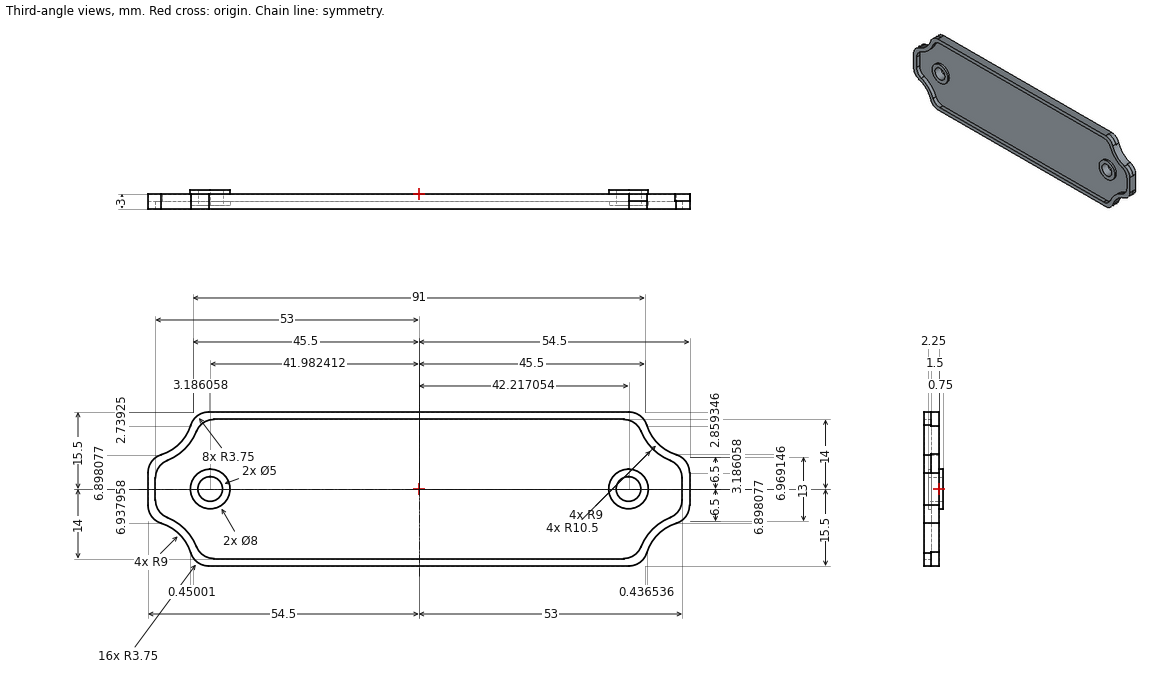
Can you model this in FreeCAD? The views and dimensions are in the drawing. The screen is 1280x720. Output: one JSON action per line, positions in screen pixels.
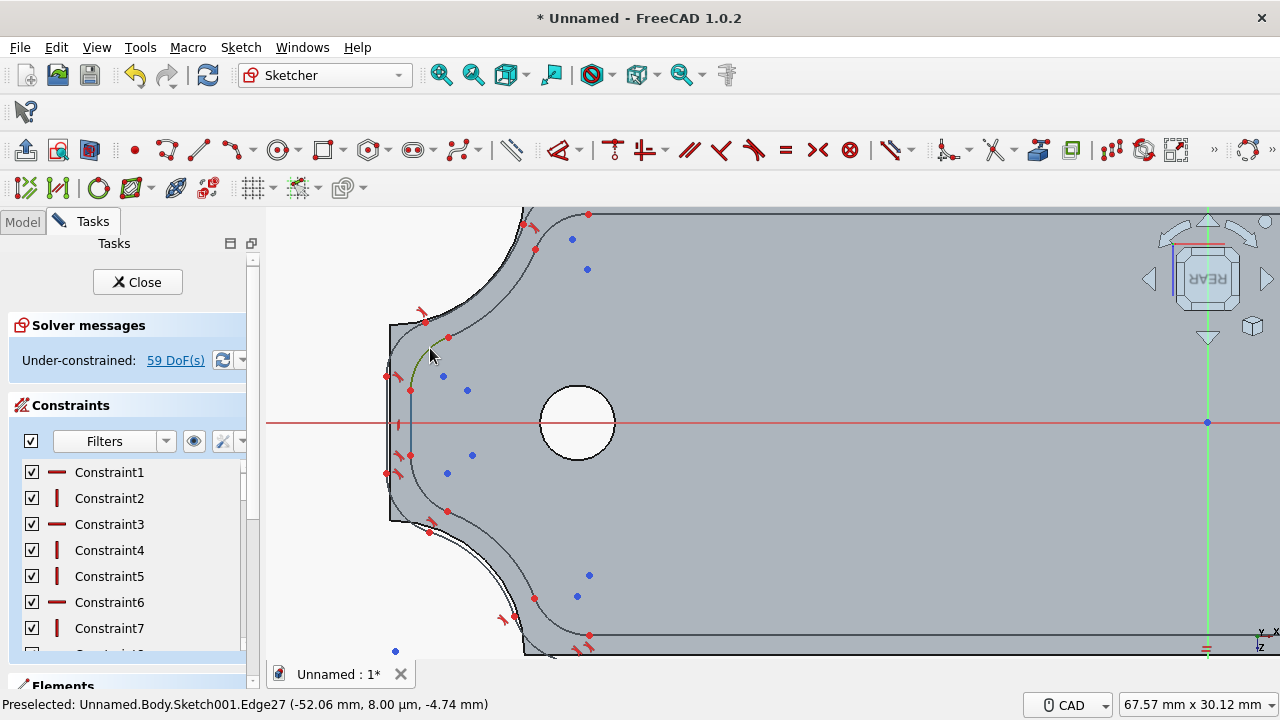
{"action": "left_click", "coordinate": [754, 150]}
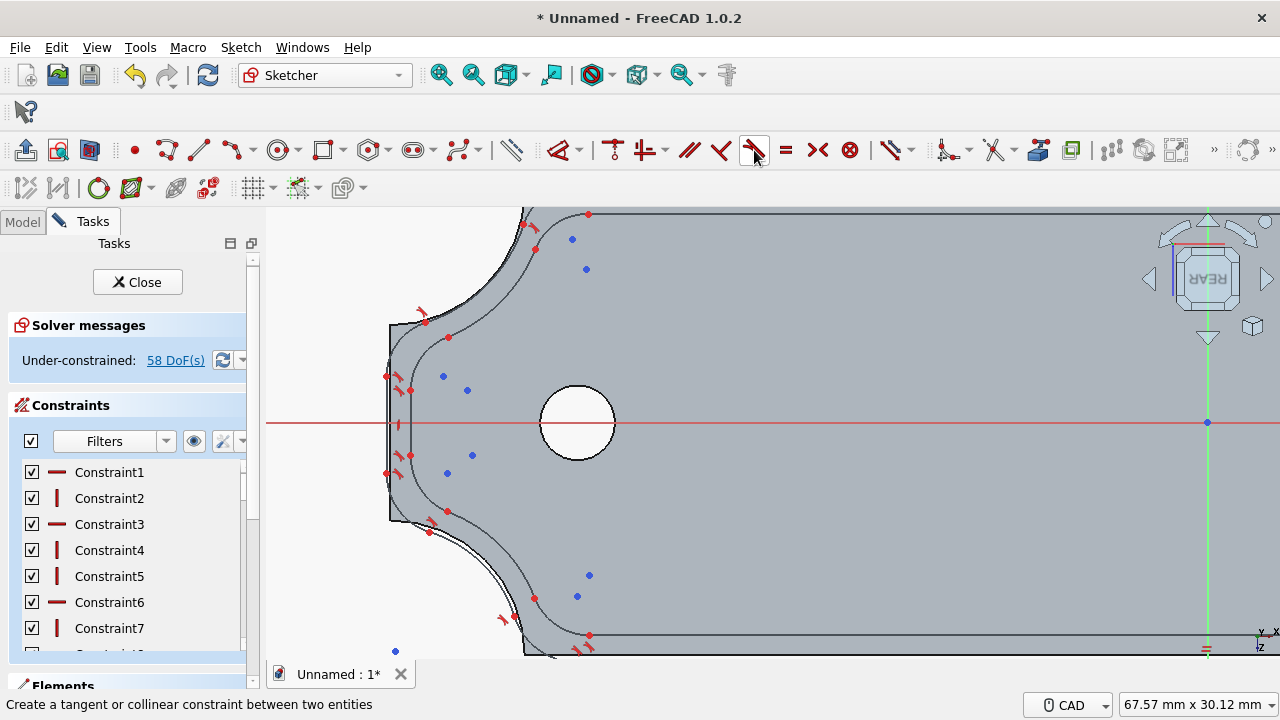
{"action": "scroll", "coordinate": [412, 439], "scroll_direction": "down", "scroll_amount": 5}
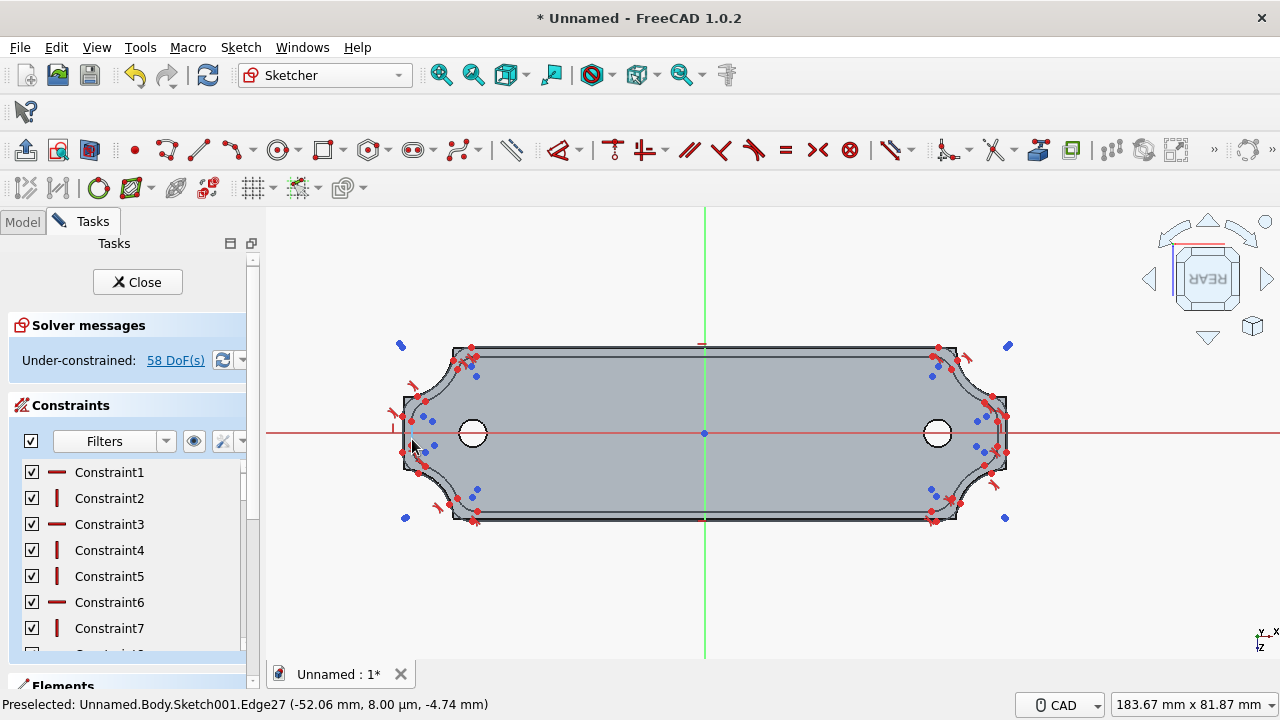
{"action": "scroll", "coordinate": [614, 357], "scroll_direction": "up", "scroll_amount": 2}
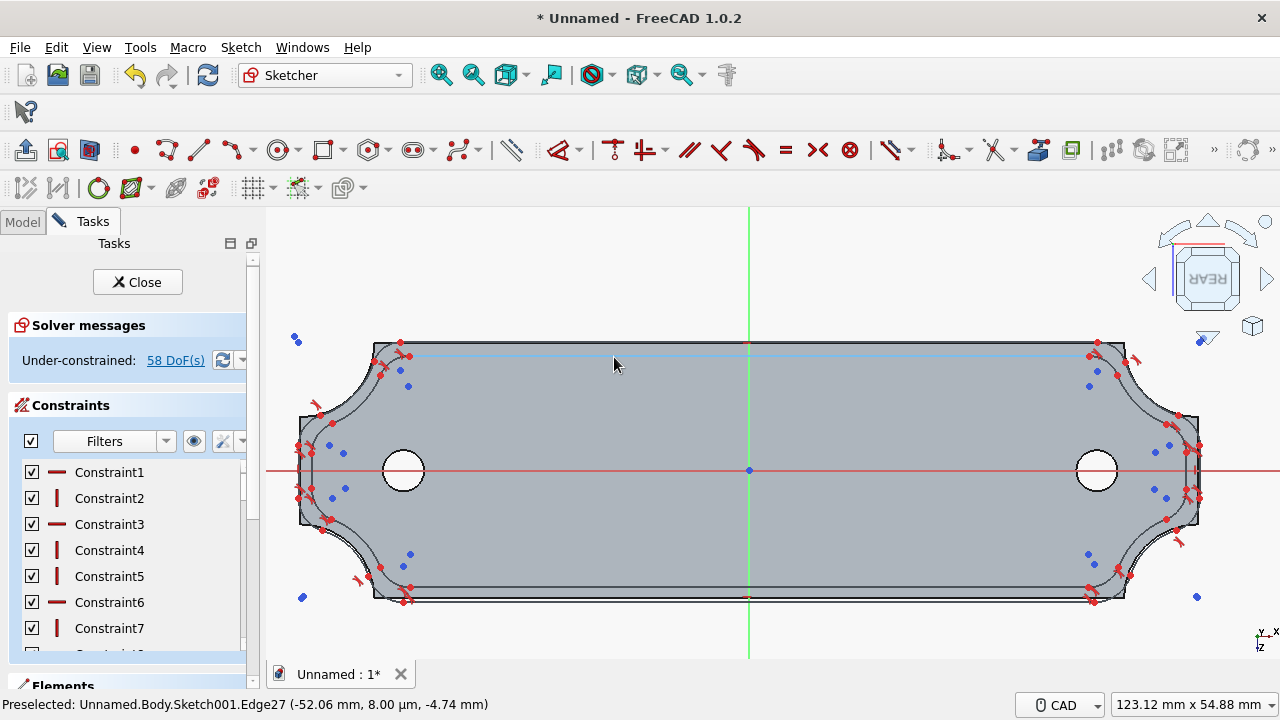
{"action": "left_click", "coordinate": [613, 356]}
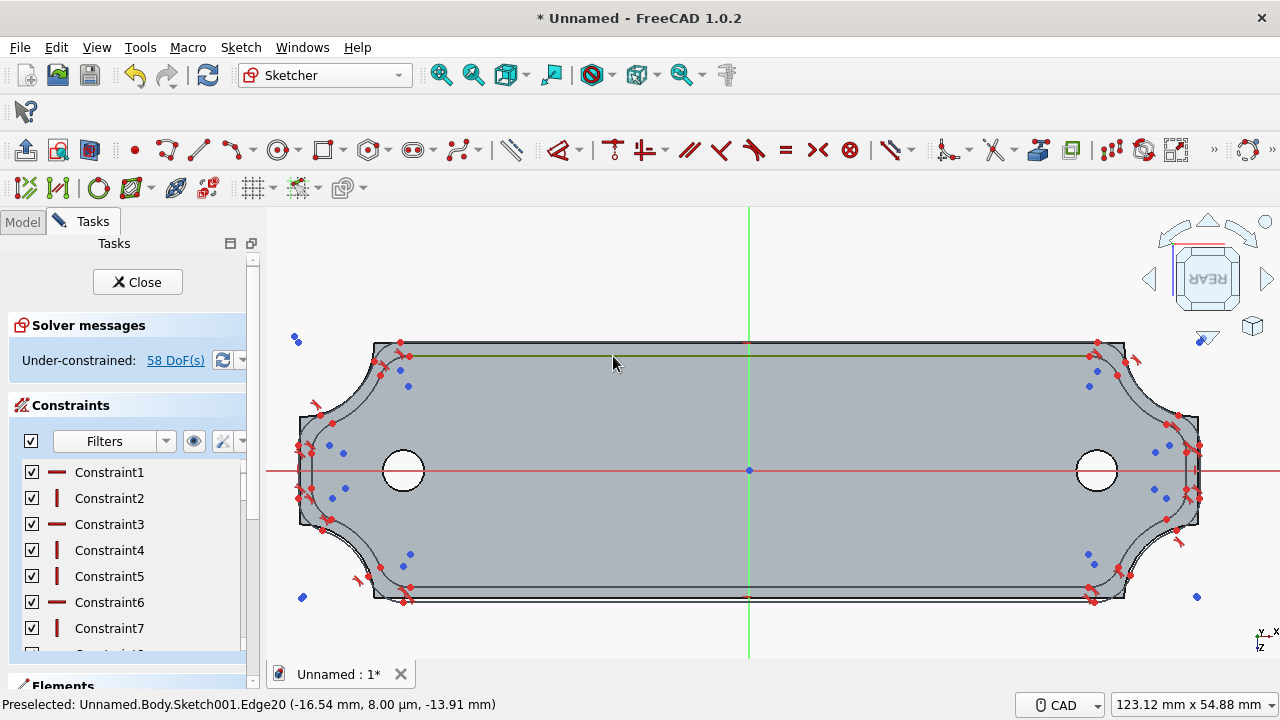
{"action": "scroll", "coordinate": [398, 358], "scroll_direction": "up", "scroll_amount": 2}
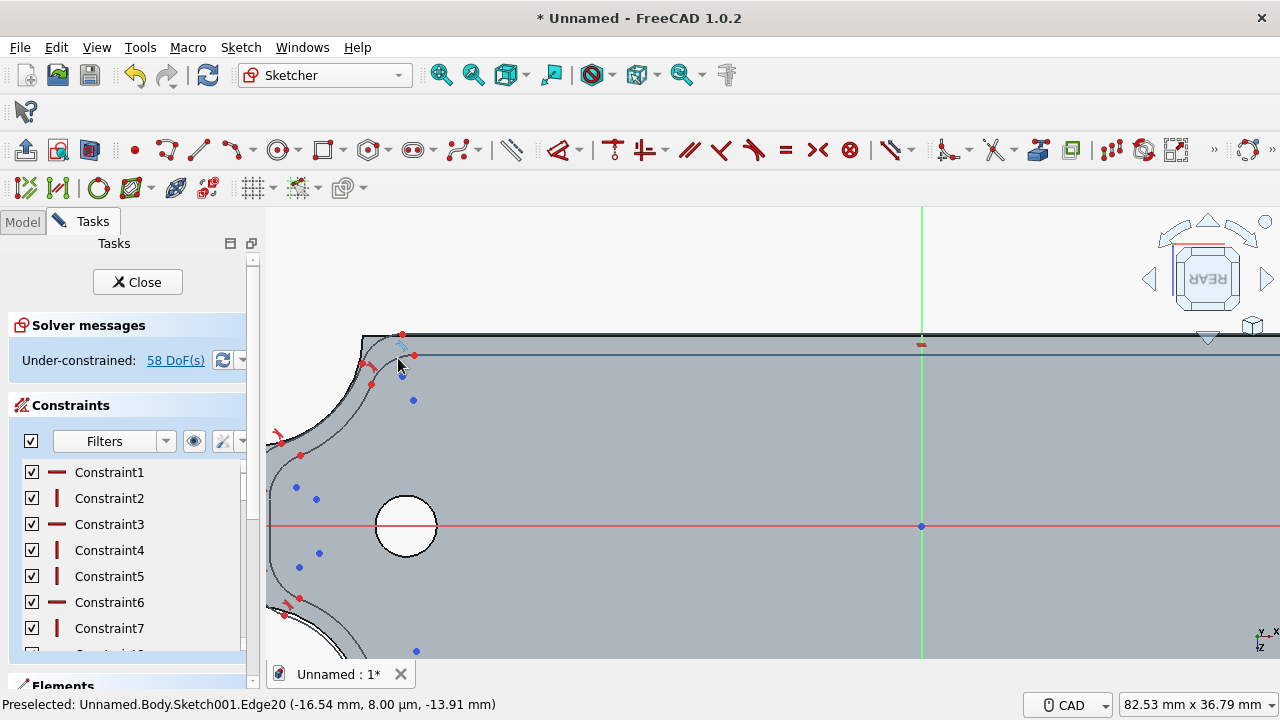
{"action": "left_click", "coordinate": [398, 358]}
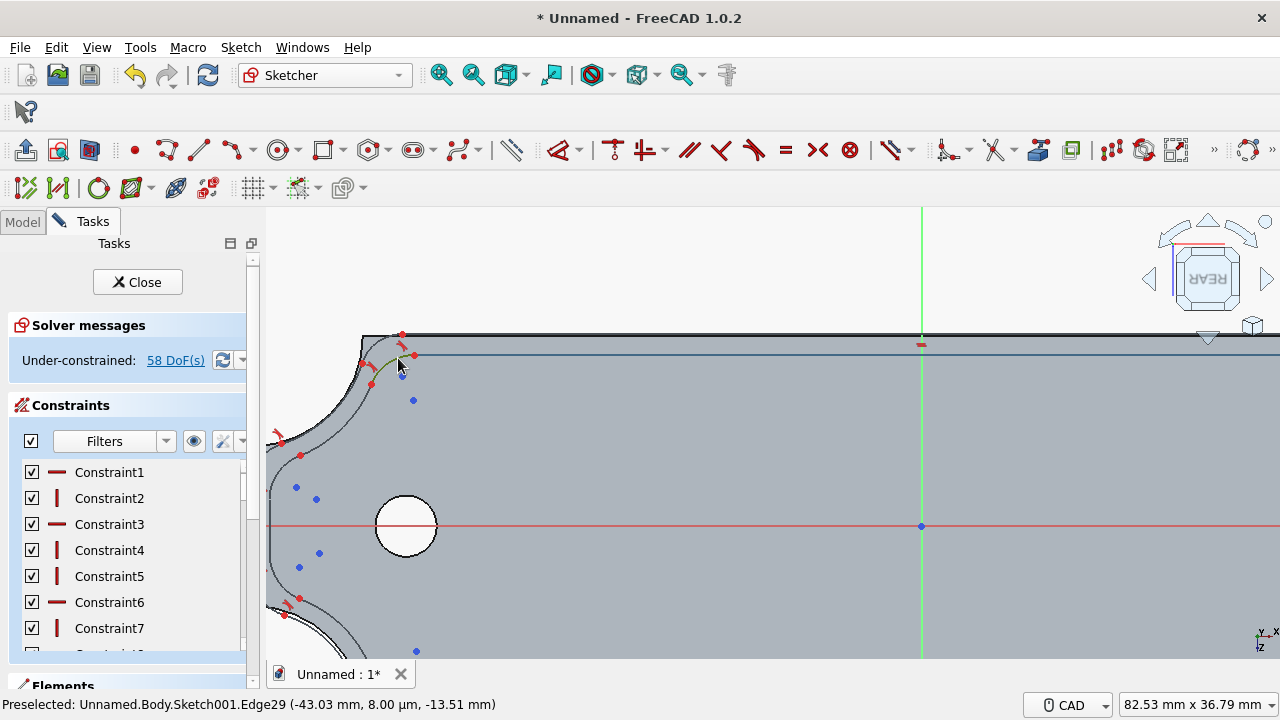
{"action": "left_click", "coordinate": [754, 150]}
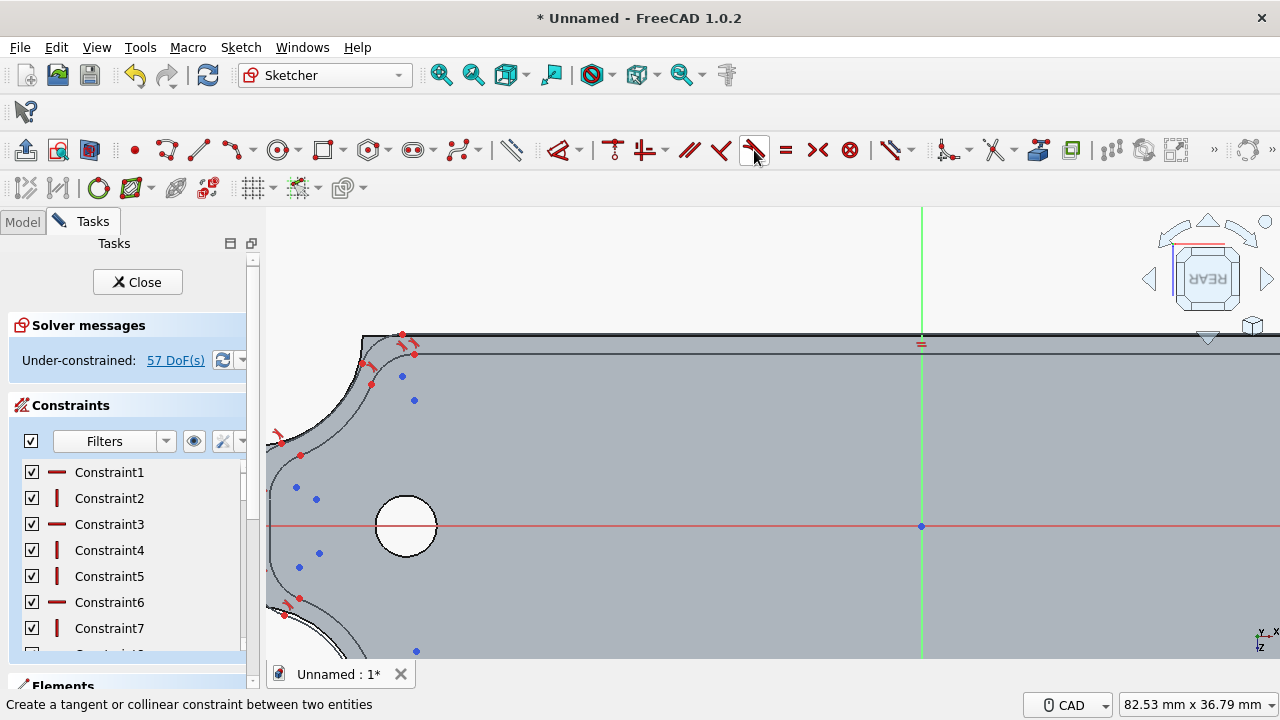
{"action": "left_click", "coordinate": [719, 354]}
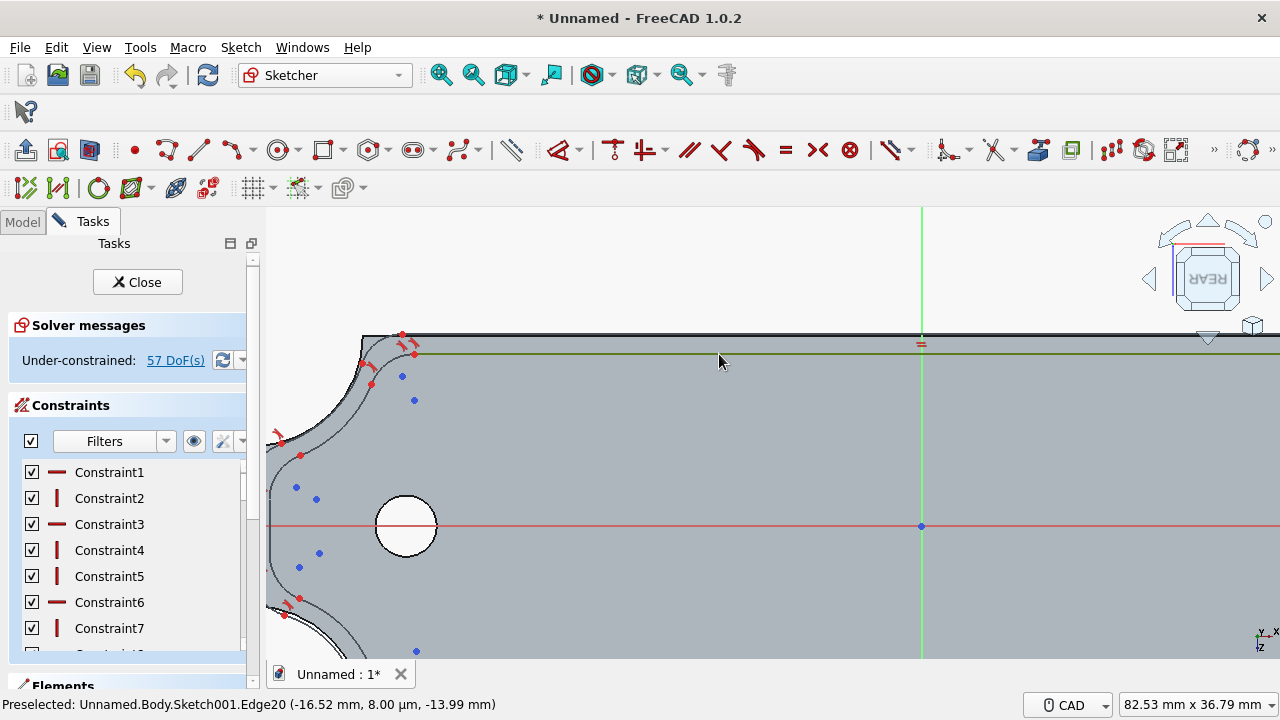
{"action": "scroll", "coordinate": [527, 357], "scroll_direction": "down", "scroll_amount": 4}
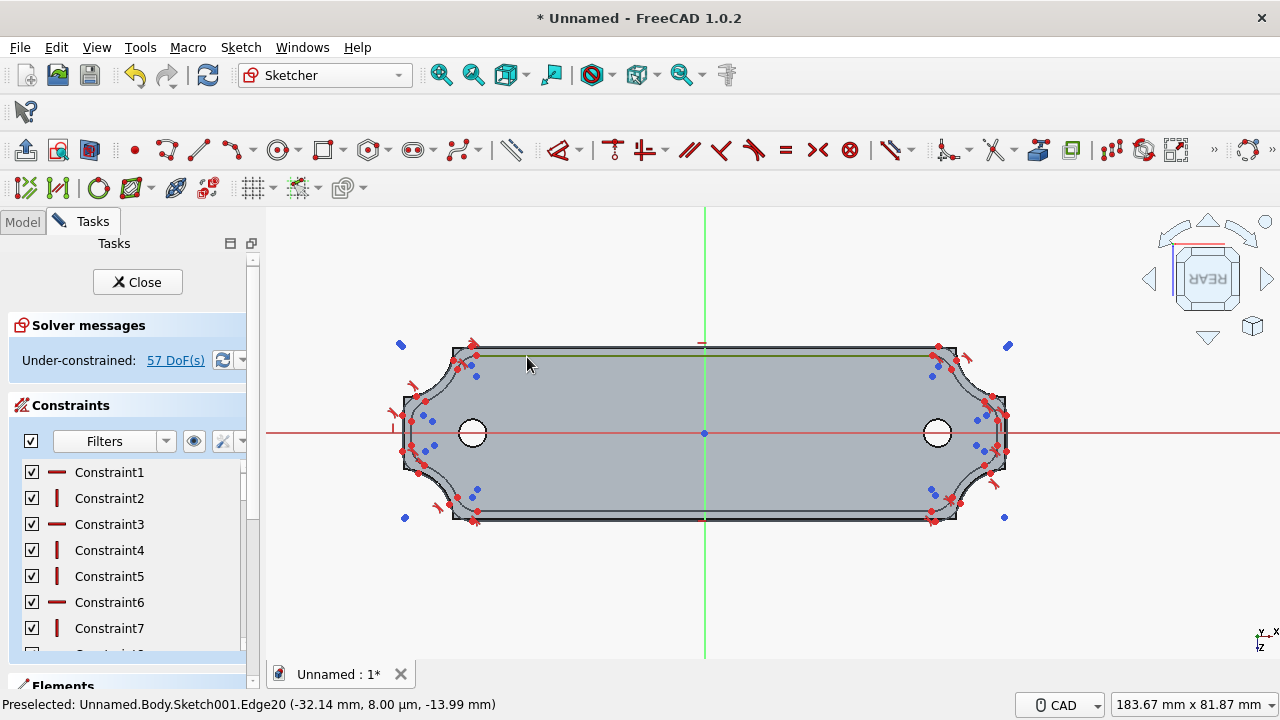
{"action": "scroll", "coordinate": [948, 363], "scroll_direction": "up", "scroll_amount": 4}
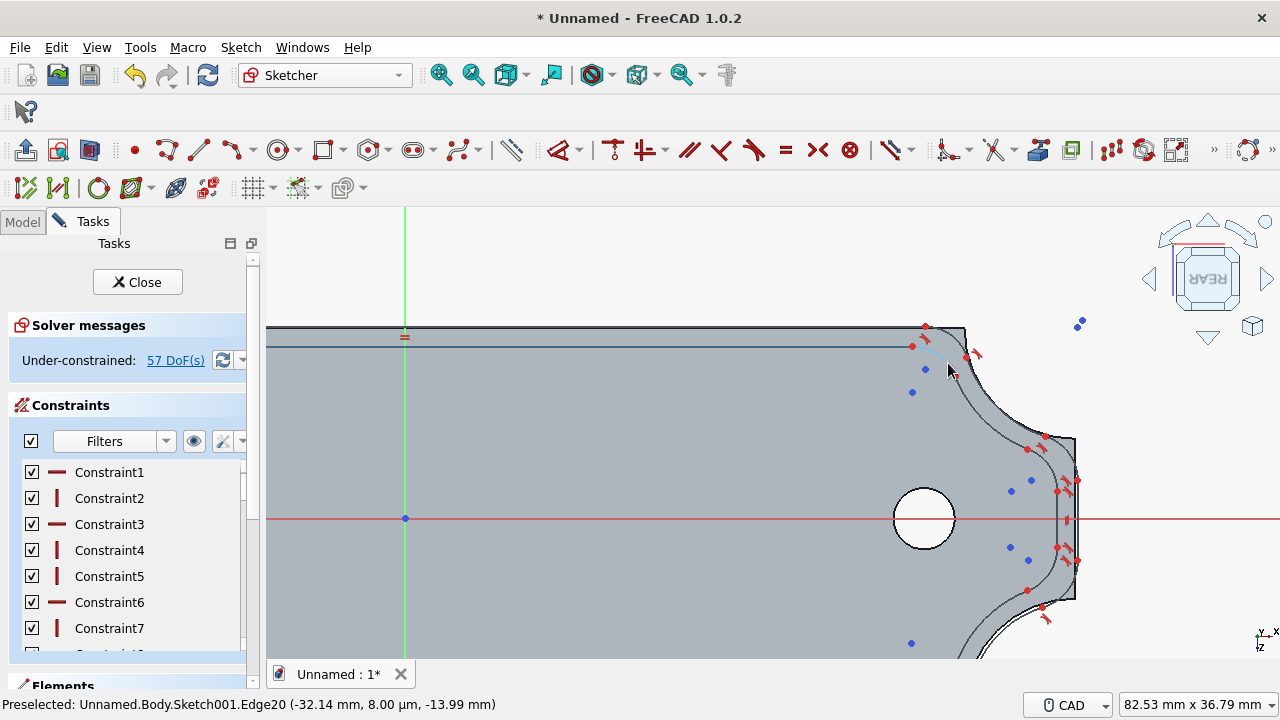
{"action": "left_click", "coordinate": [947, 362]}